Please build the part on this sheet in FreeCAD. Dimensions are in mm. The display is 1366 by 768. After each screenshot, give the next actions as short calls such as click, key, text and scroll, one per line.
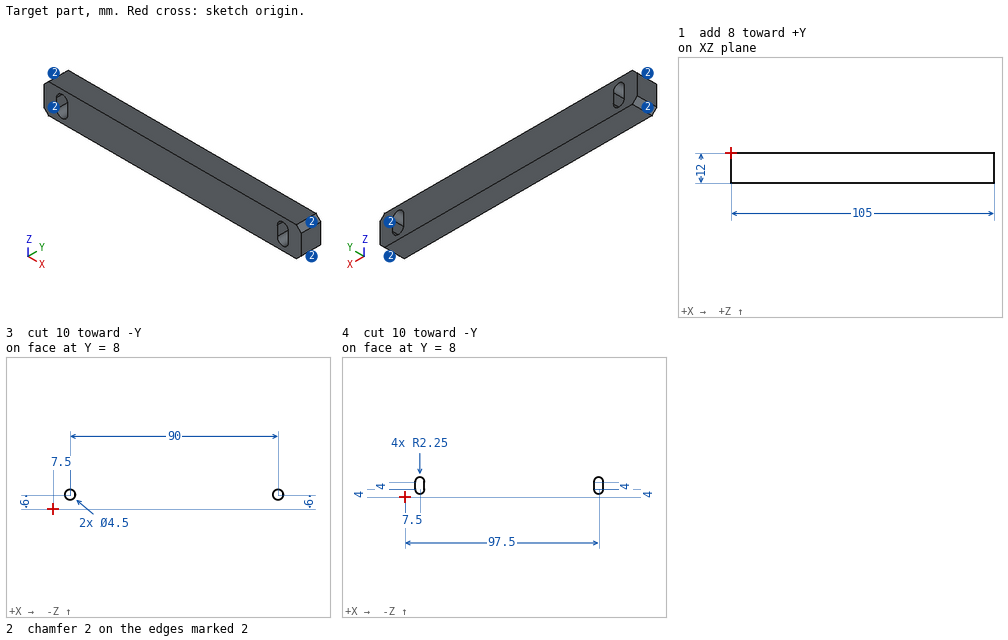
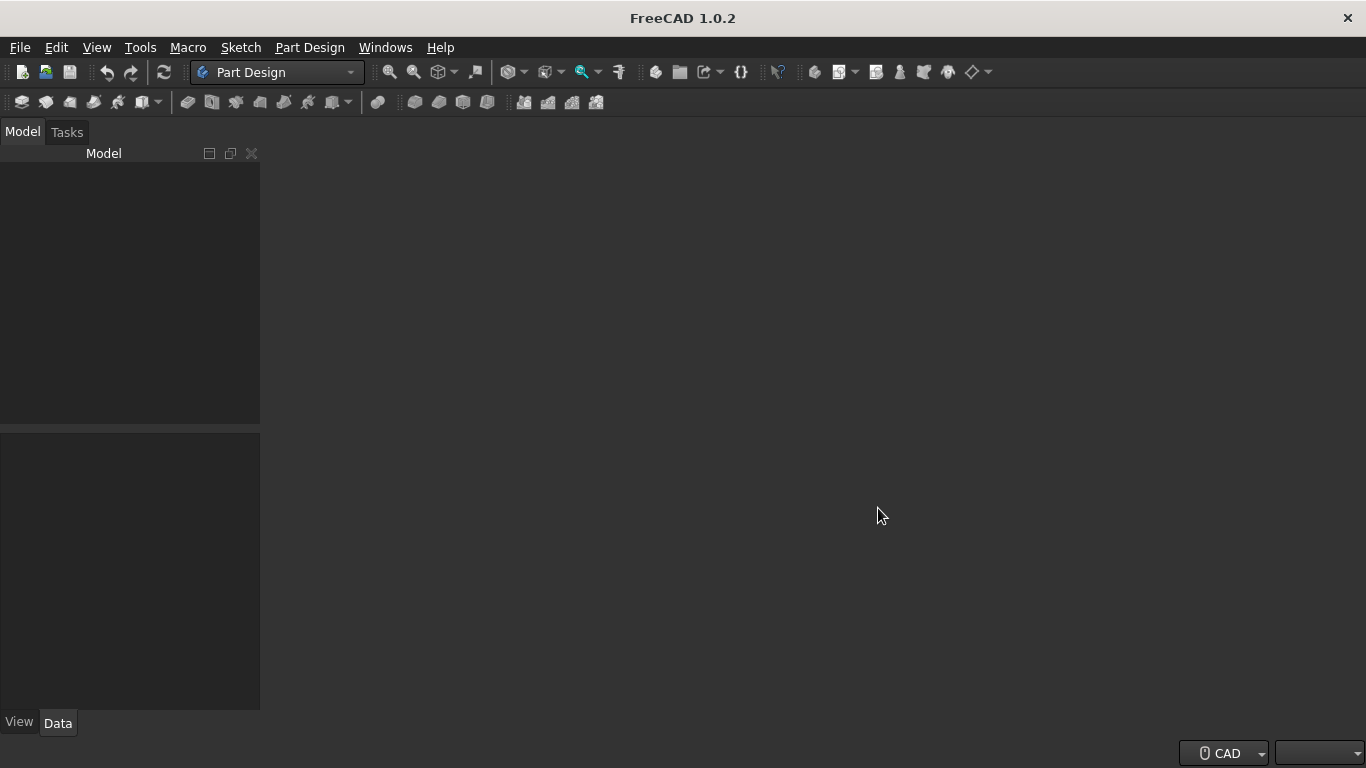
click(22, 72)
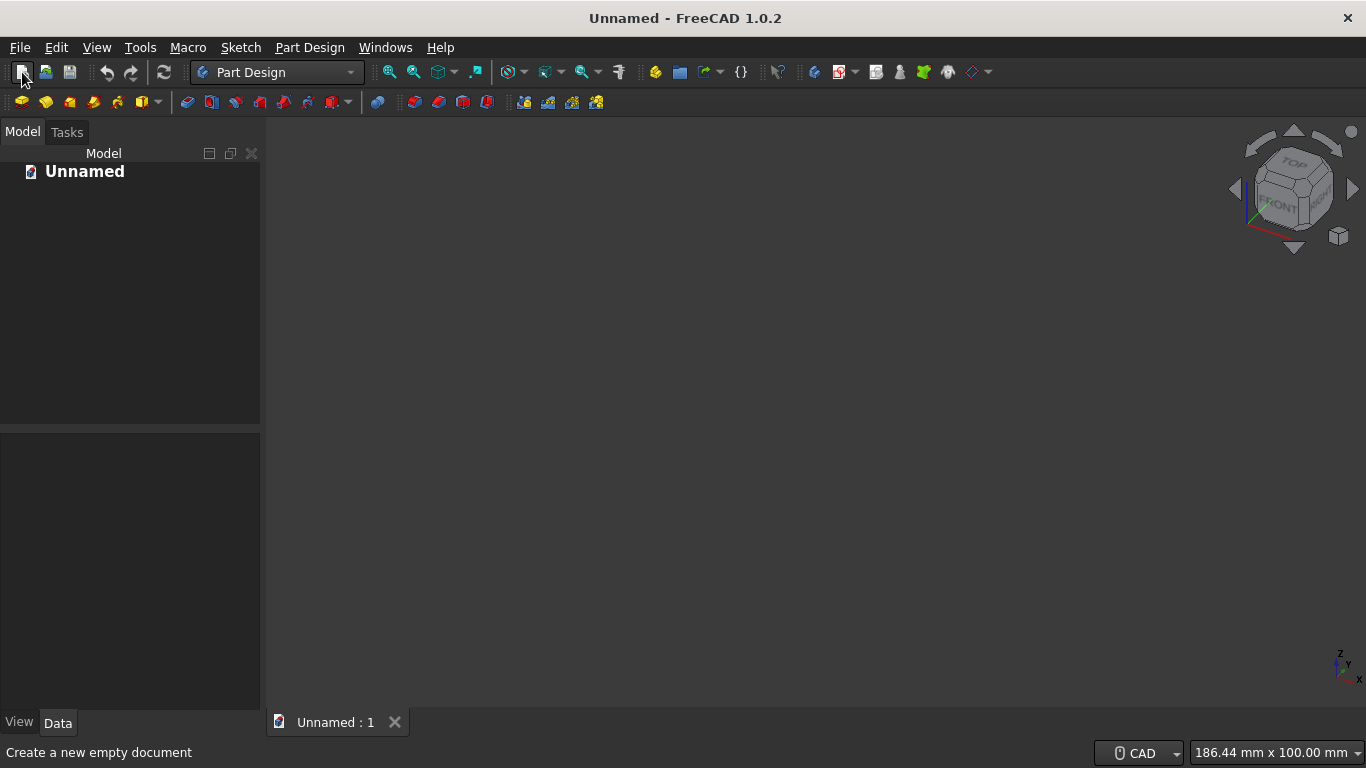
click(840, 72)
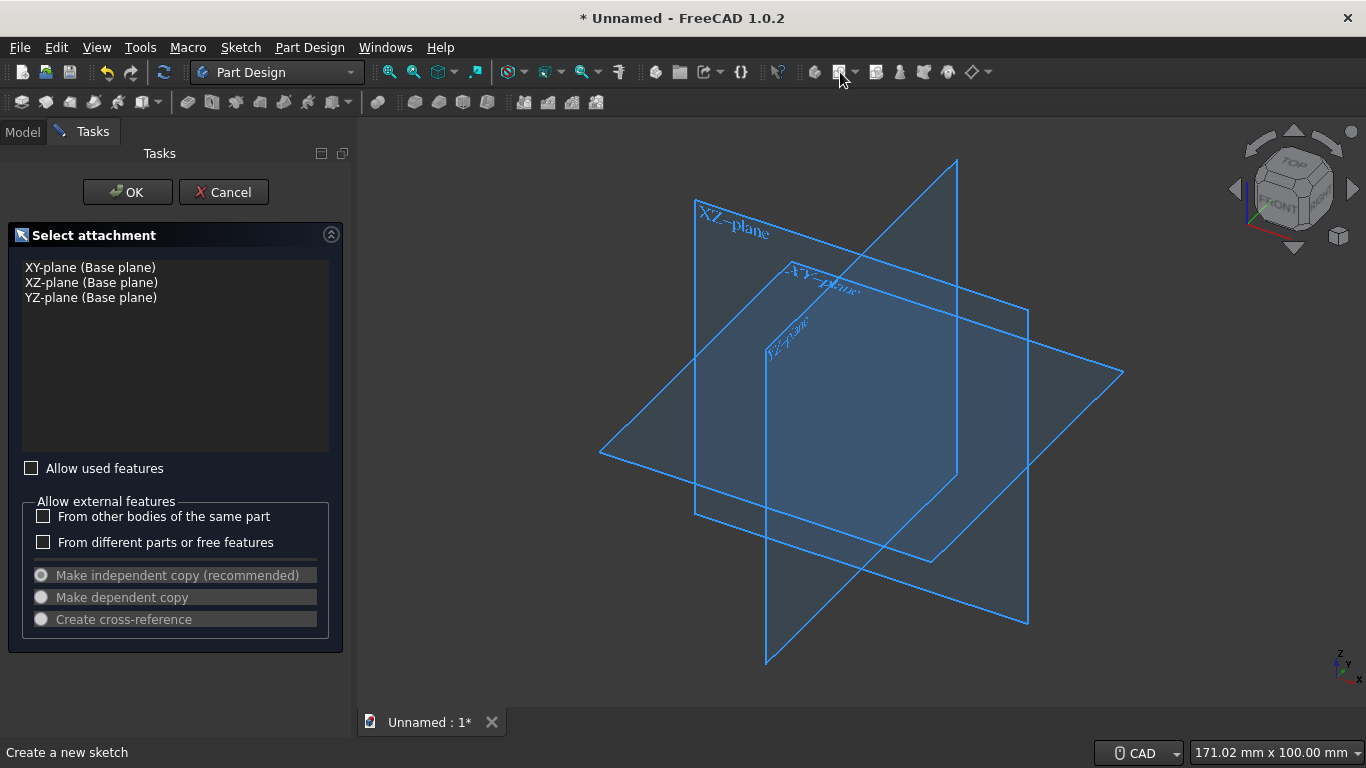
click(82, 282)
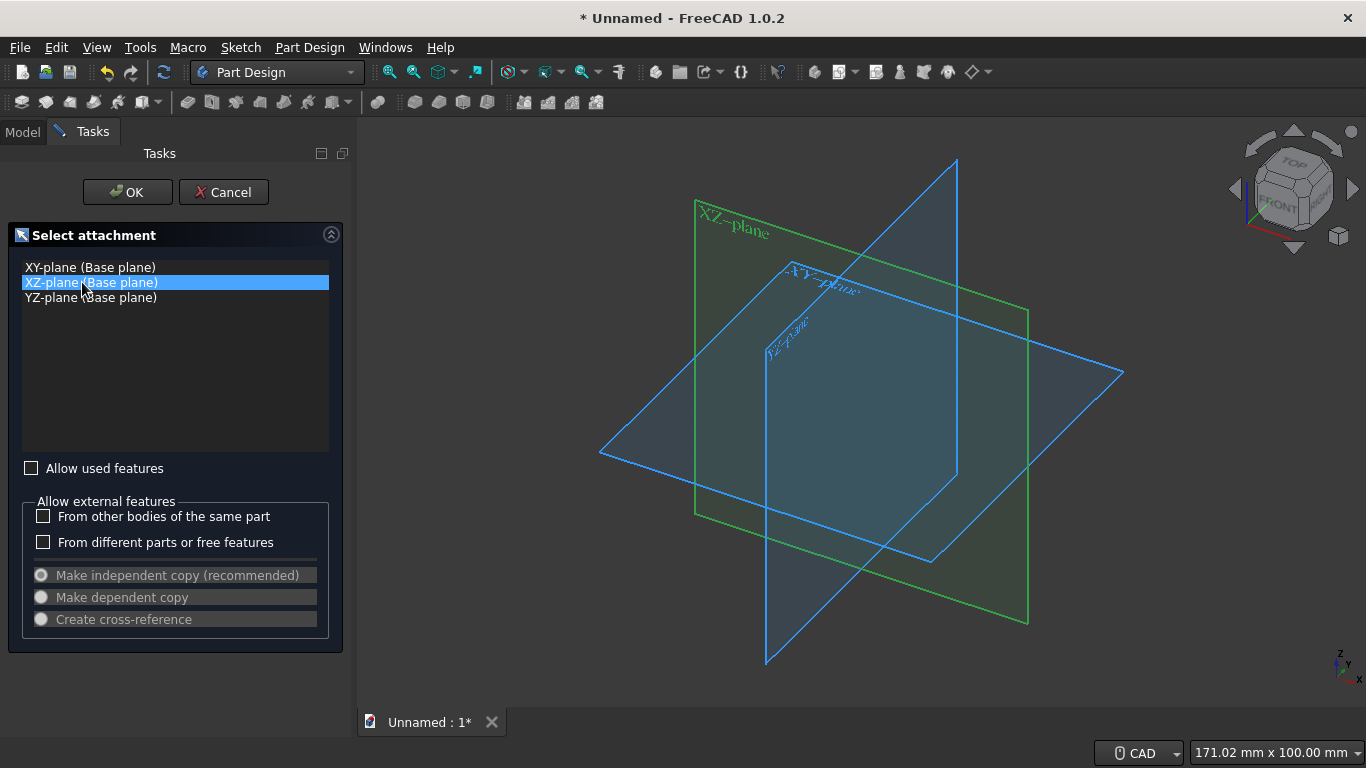
click(128, 192)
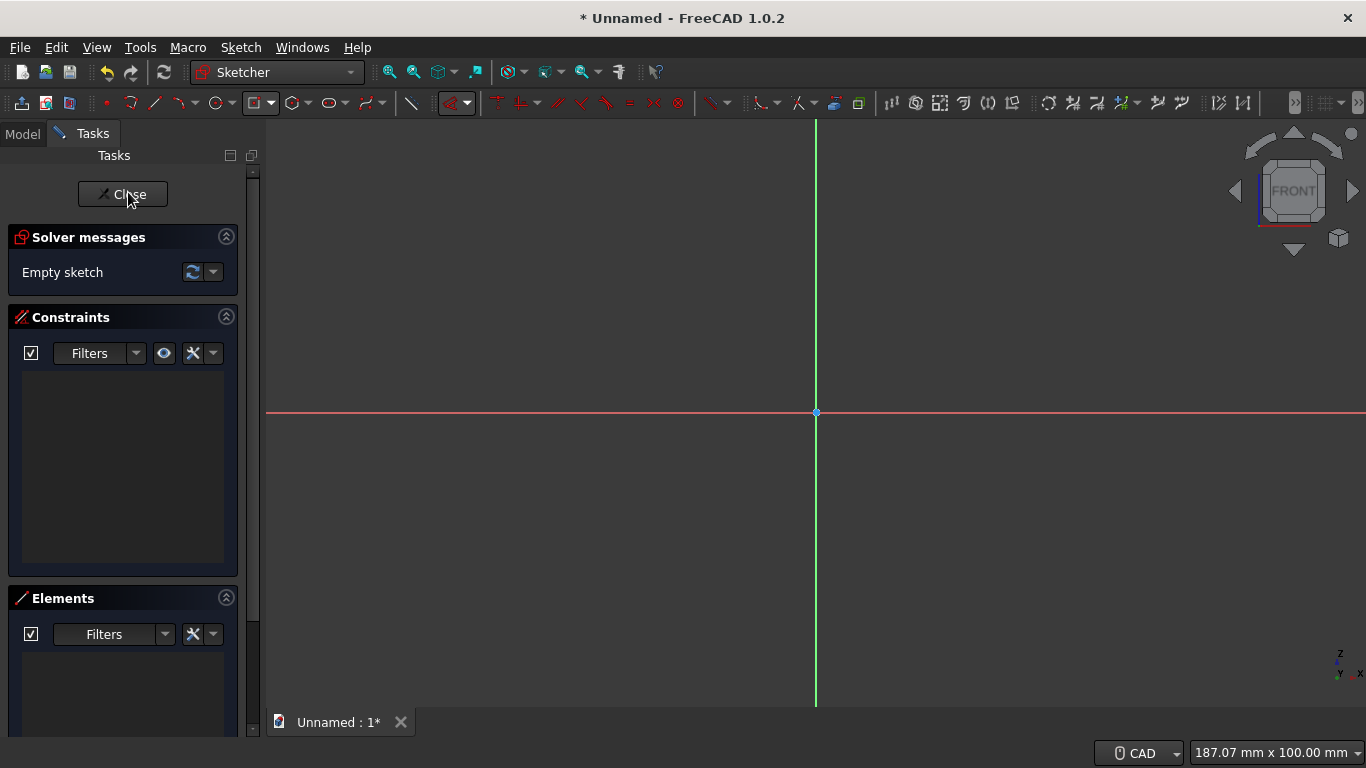
scroll(294, 341, down, 2)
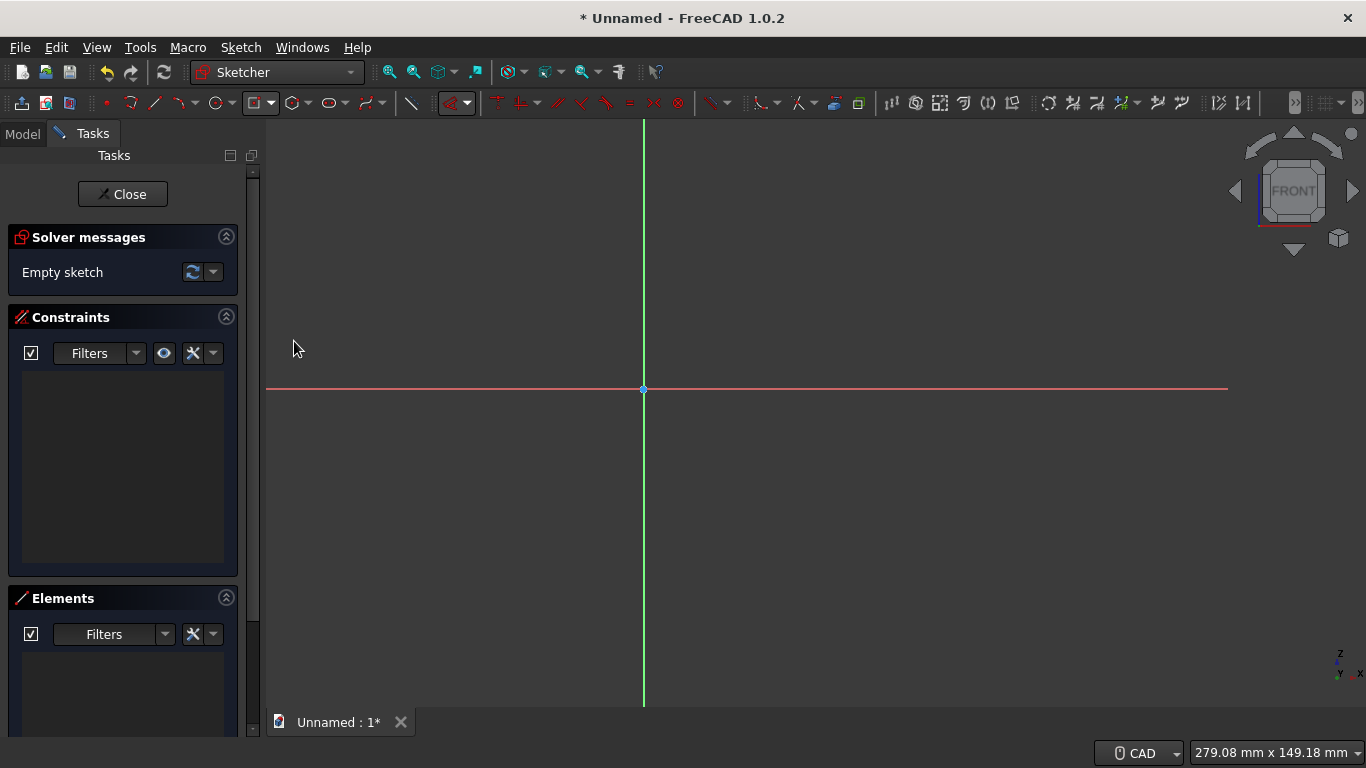
scroll(1061, 413, up, 2)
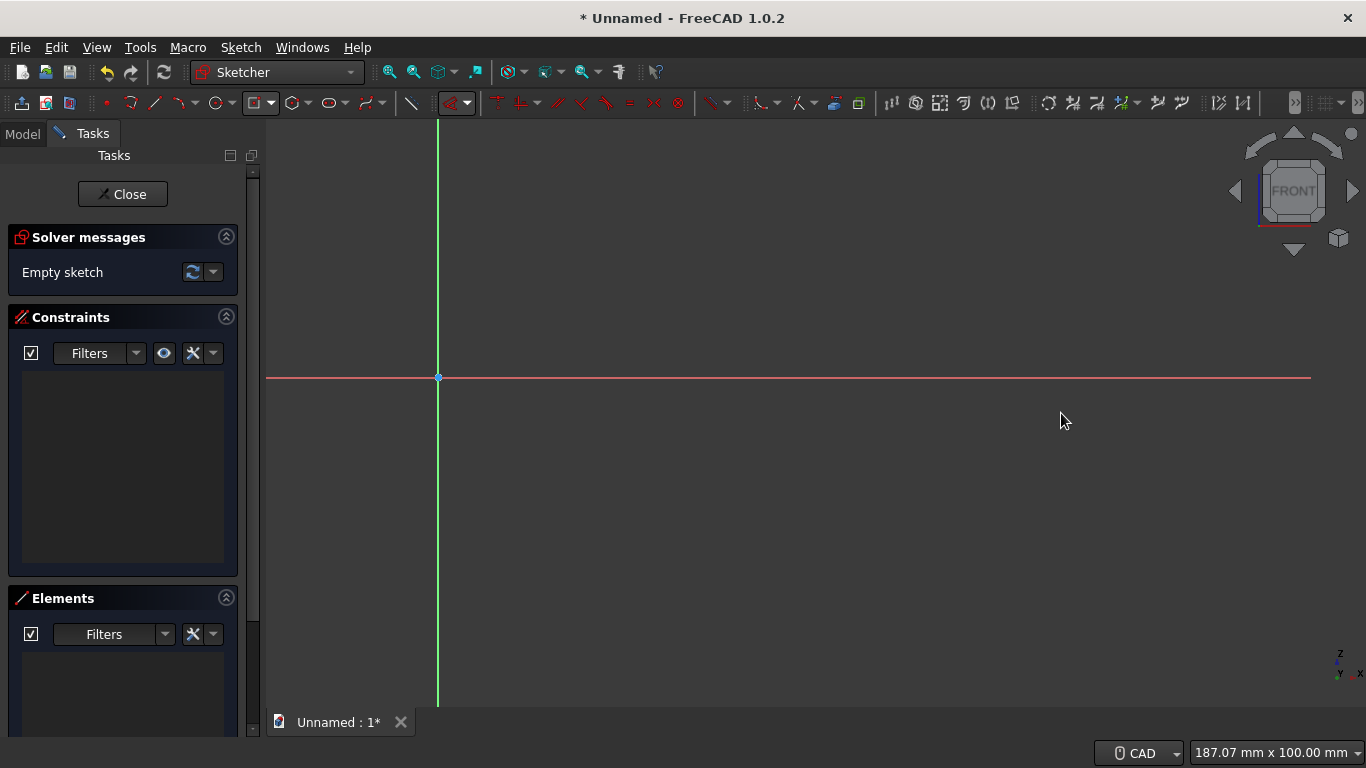
key(g)
key(r)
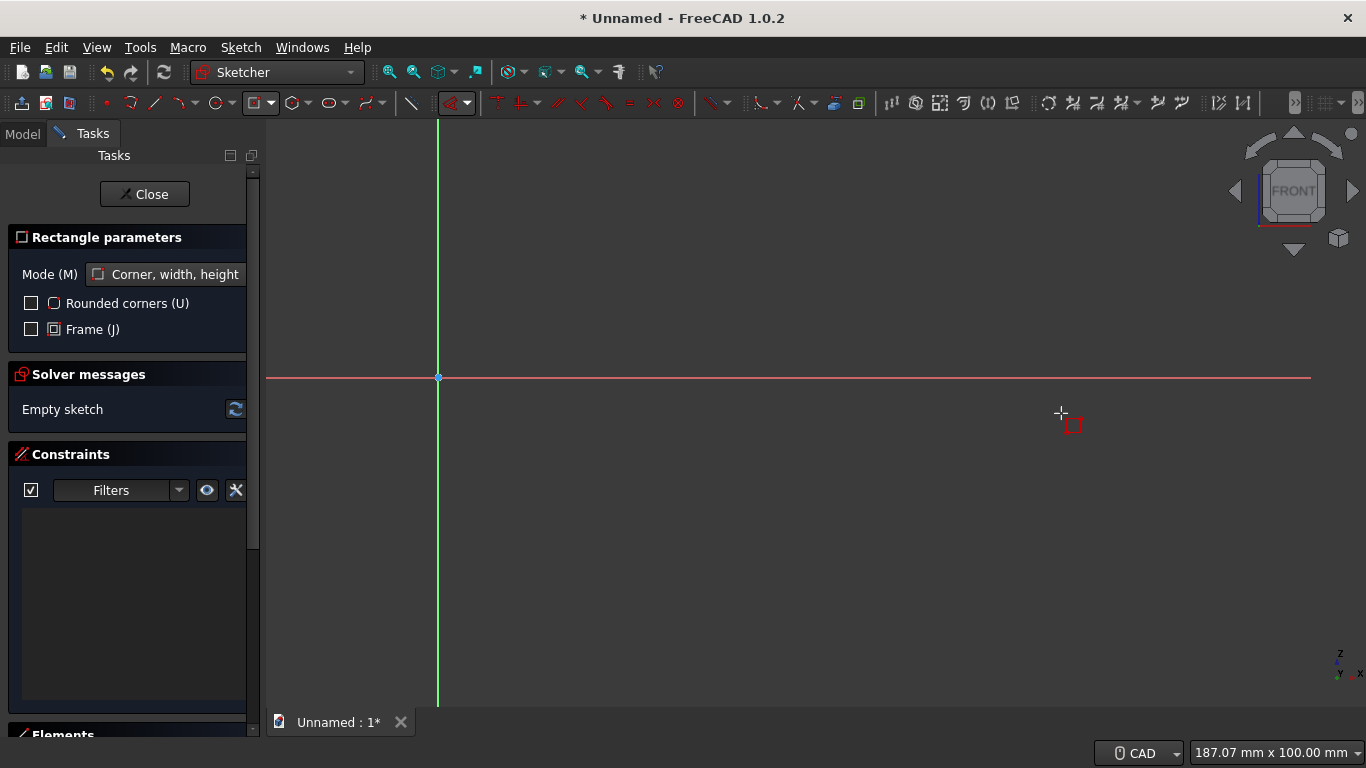
click(438, 378)
click(1056, 448)
key(Escape)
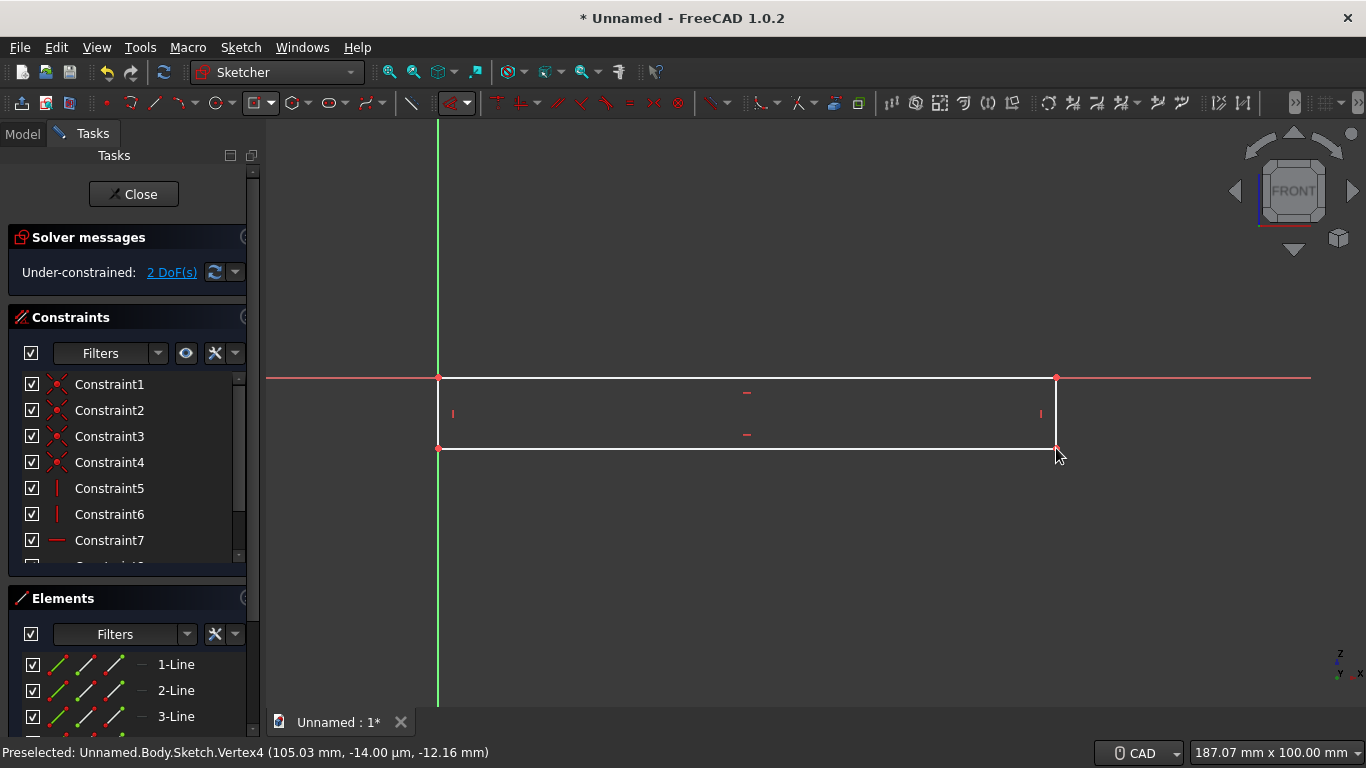
click(450, 104)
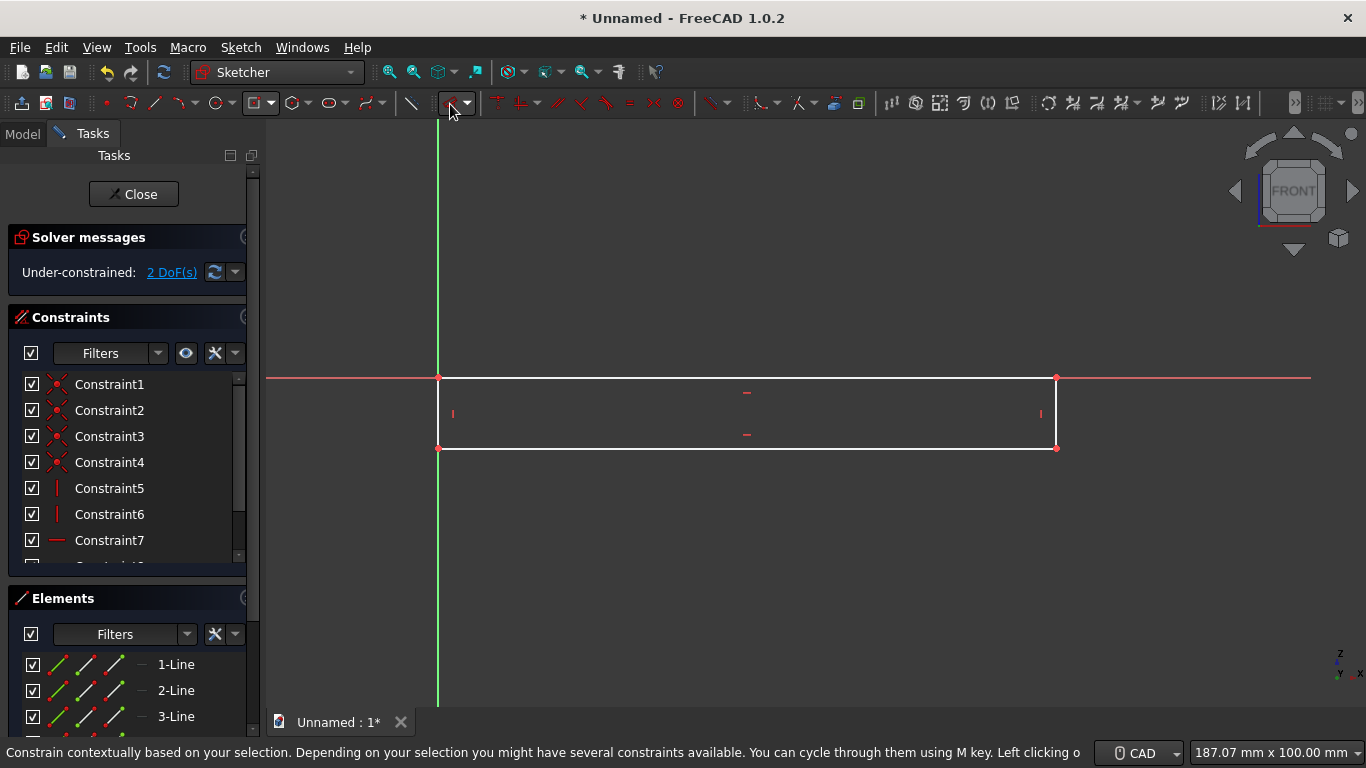
click(438, 399)
click(404, 413)